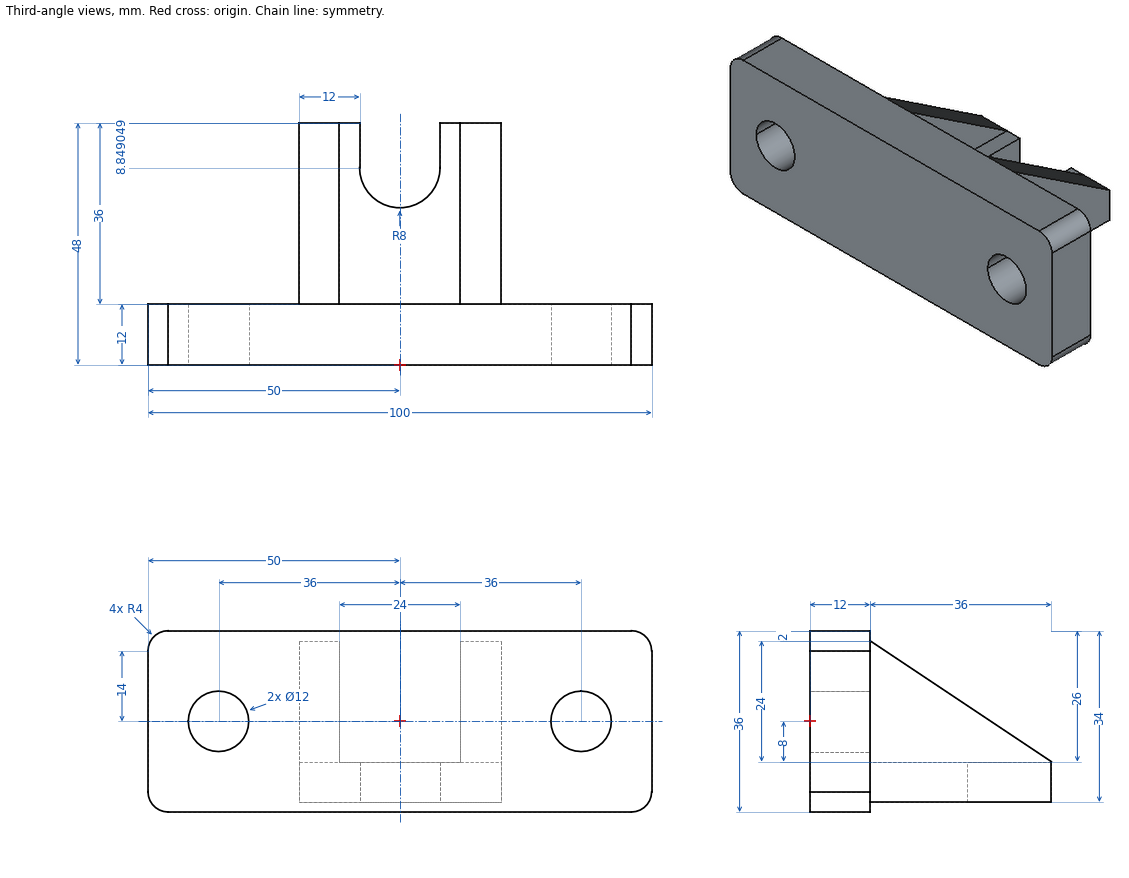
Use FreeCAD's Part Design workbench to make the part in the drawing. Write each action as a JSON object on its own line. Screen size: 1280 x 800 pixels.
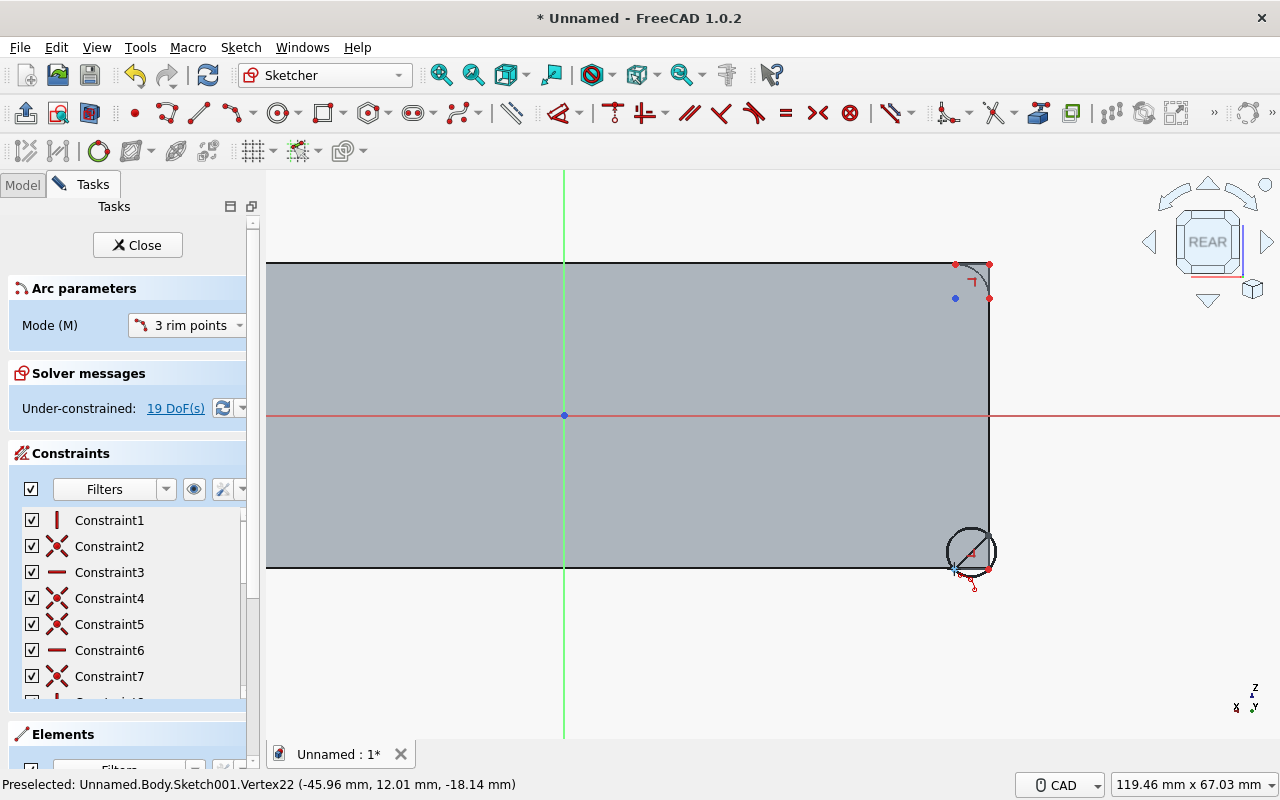
{"action": "scroll", "coordinate": [979, 558], "scroll_direction": "up", "scroll_amount": 3}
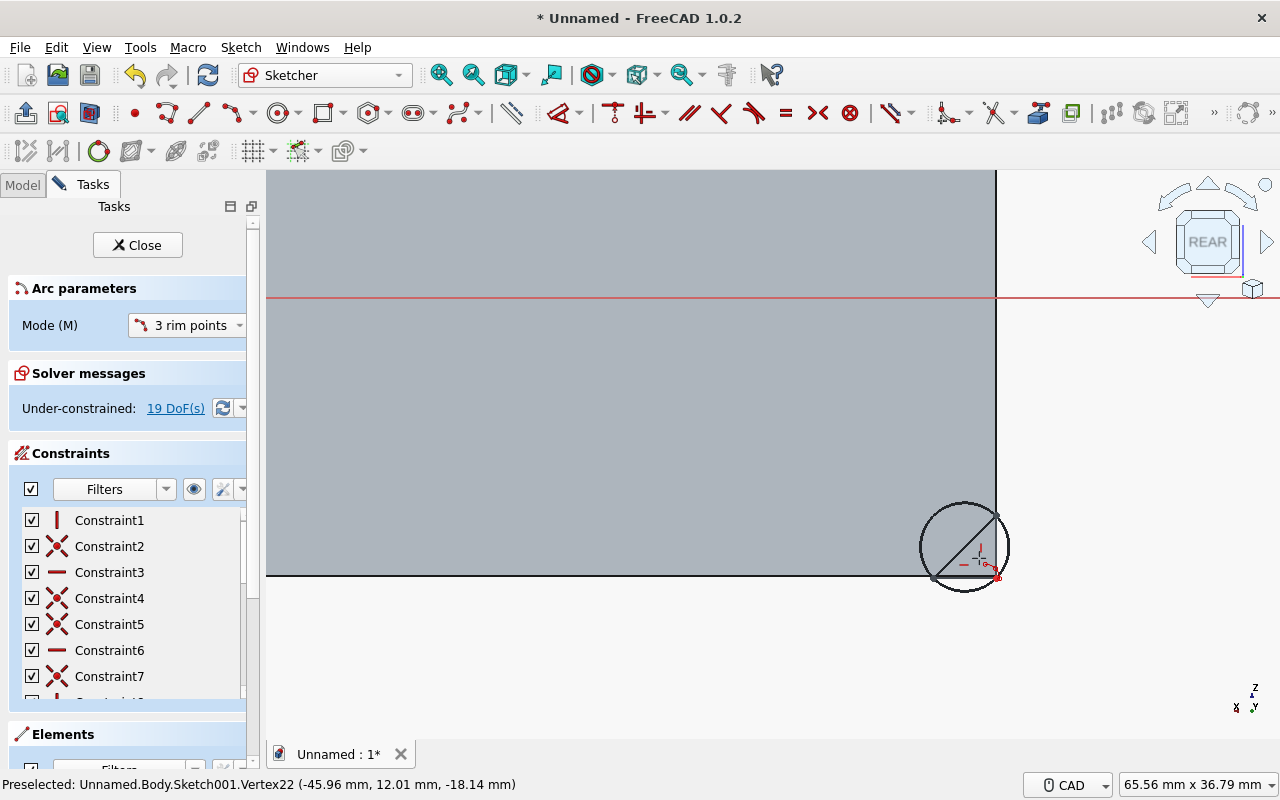
{"action": "left_click", "coordinate": [978, 558]}
{"action": "key", "text": "Escape"}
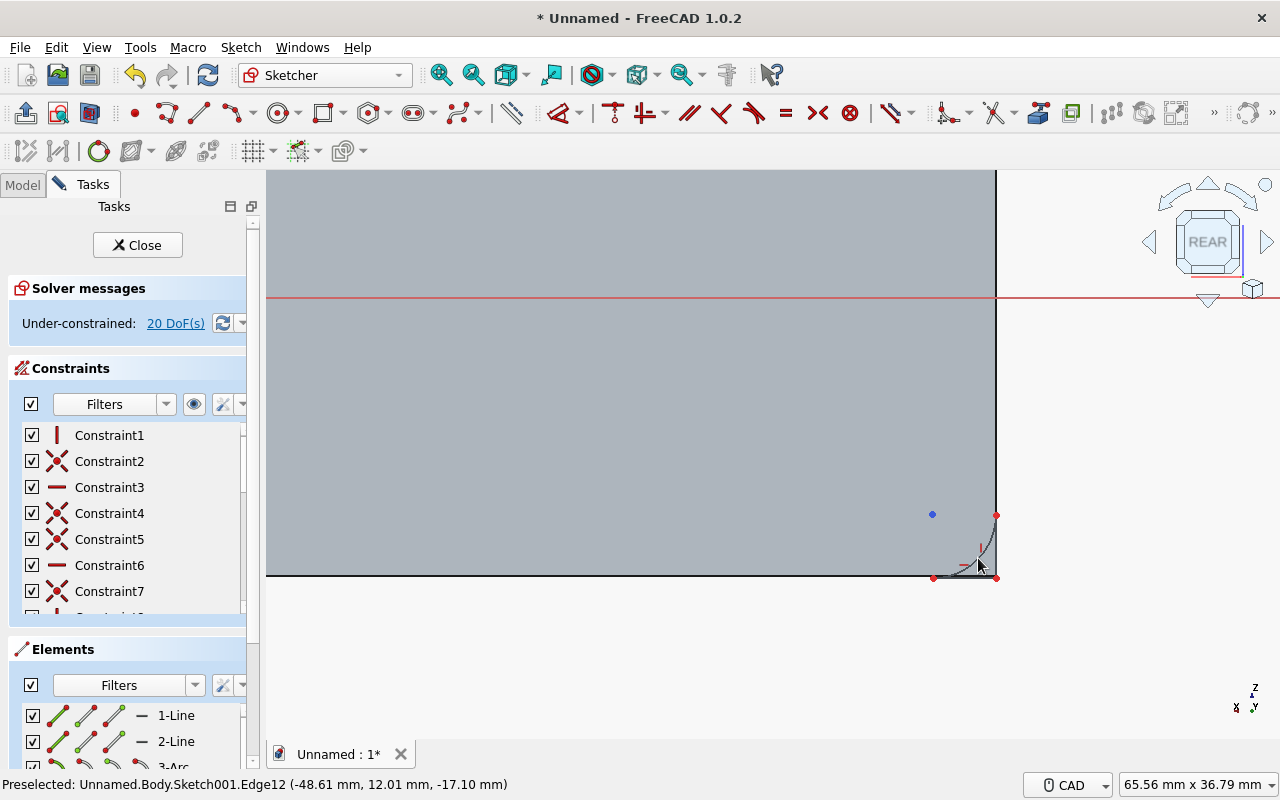
{"action": "scroll", "coordinate": [985, 546], "scroll_direction": "down", "scroll_amount": 5}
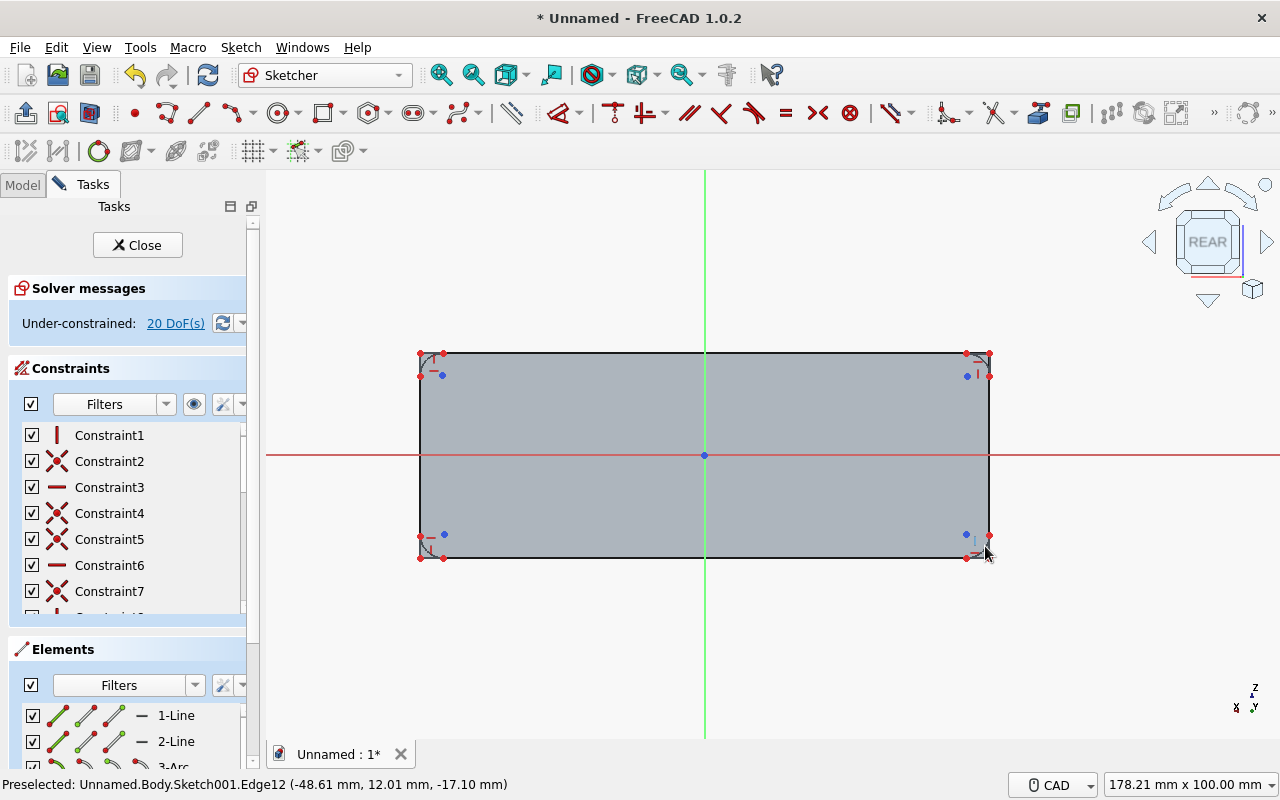
{"action": "scroll", "coordinate": [990, 361], "scroll_direction": "up", "scroll_amount": 6}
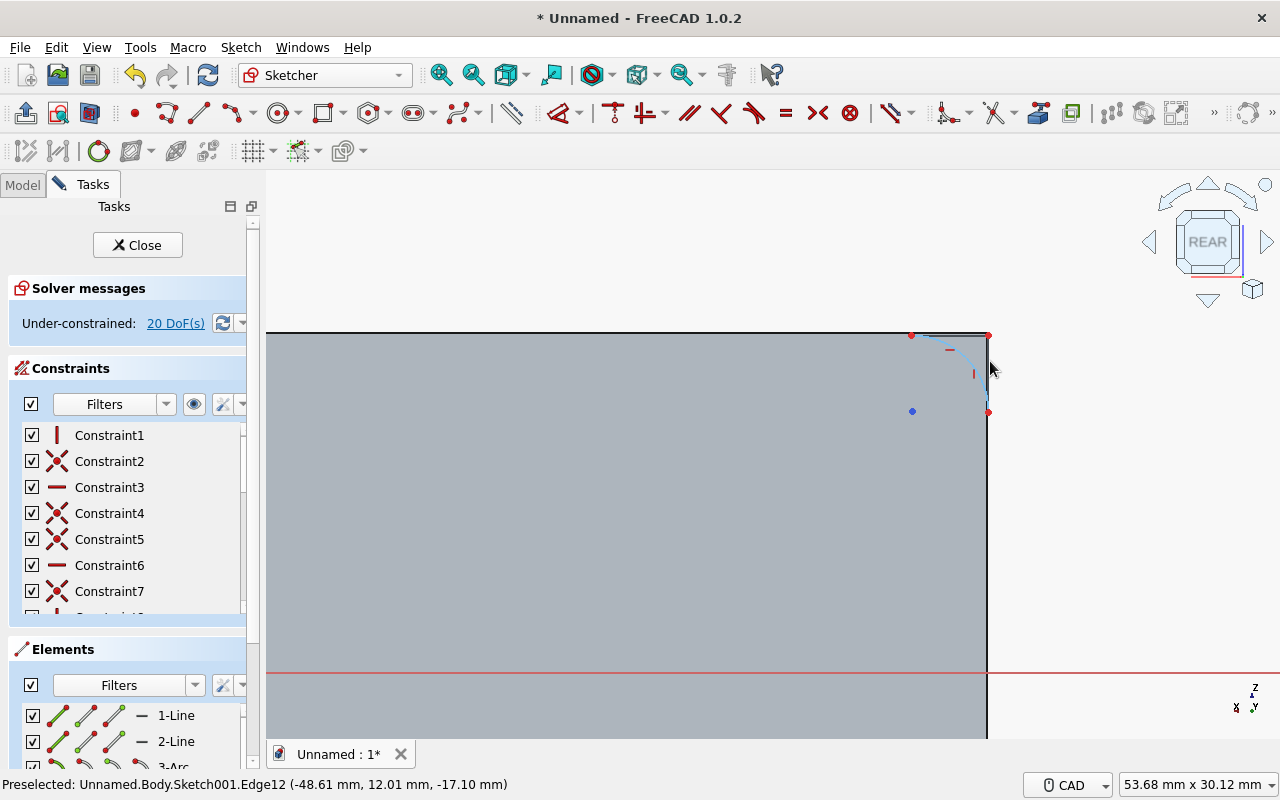
{"action": "left_click", "coordinate": [988, 359]}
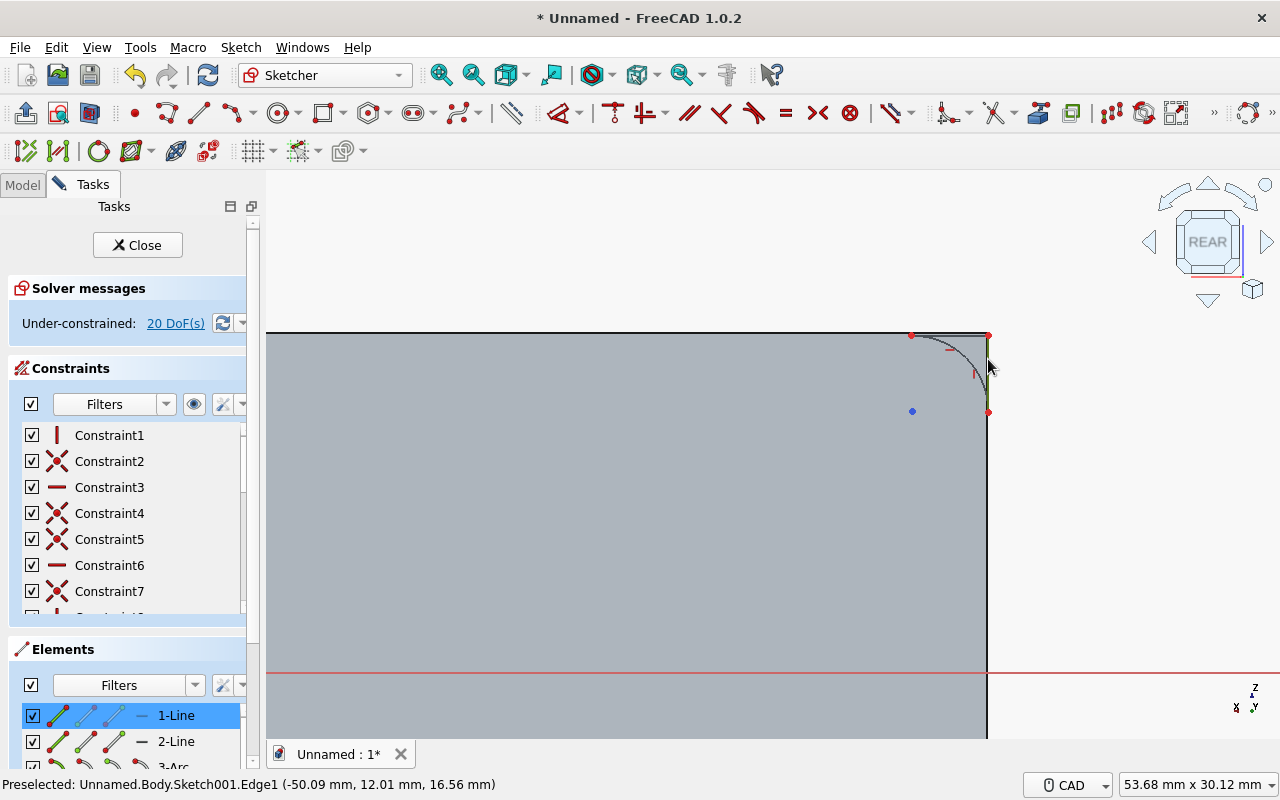
{"action": "left_click", "coordinate": [966, 358]}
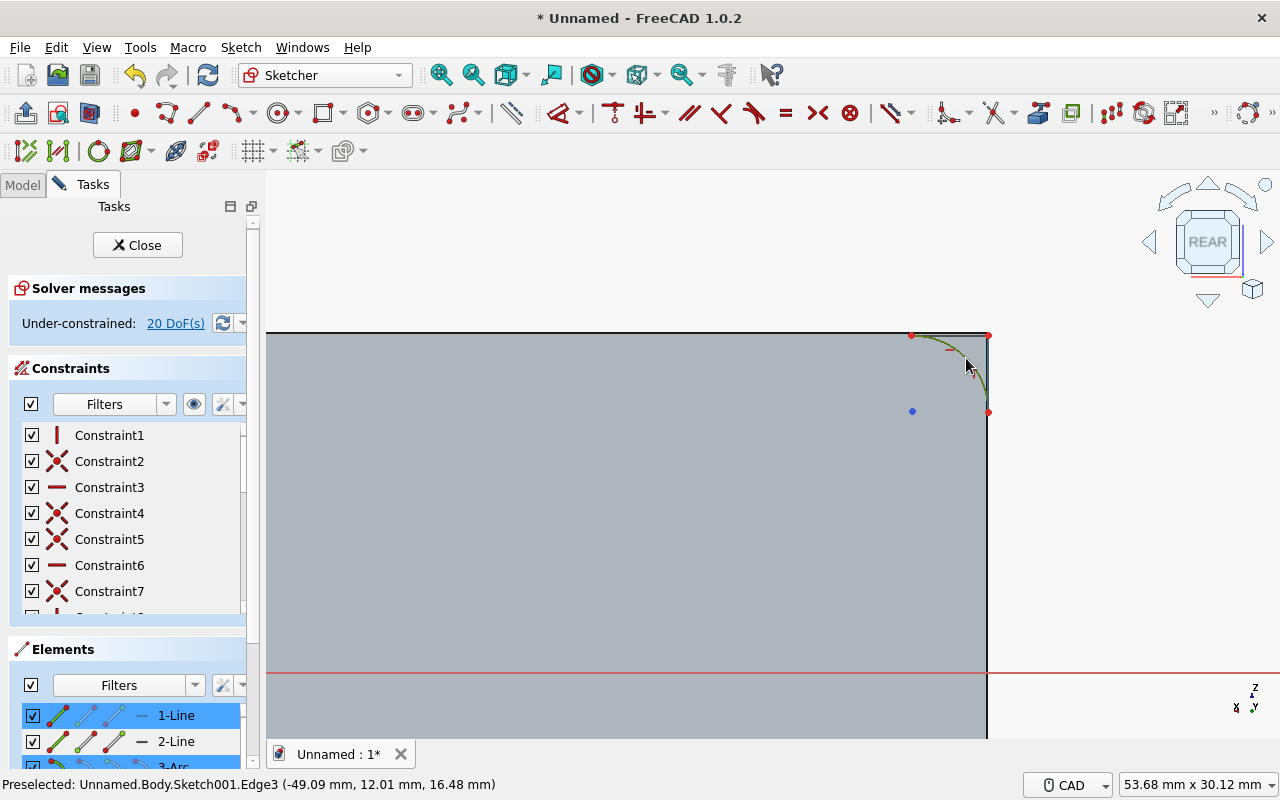
{"action": "left_click", "coordinate": [754, 114]}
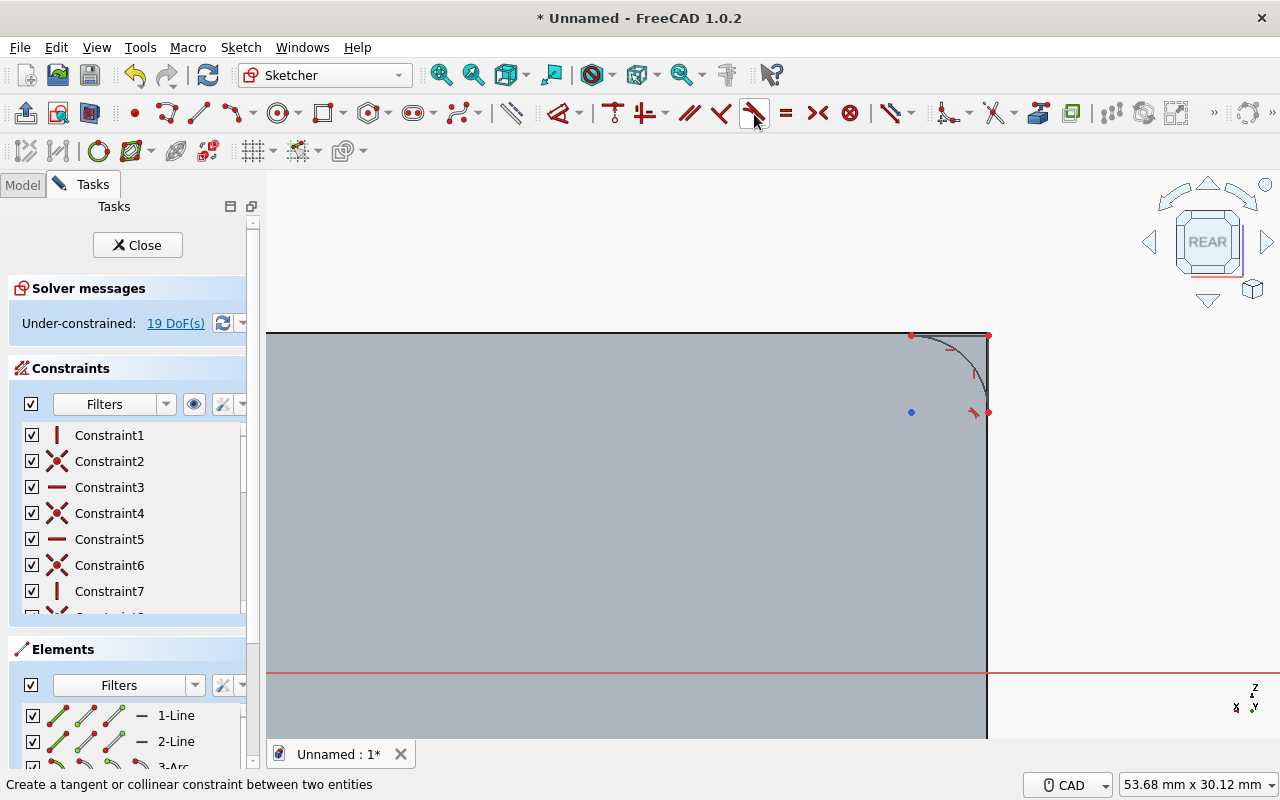
{"action": "left_click", "coordinate": [965, 336]}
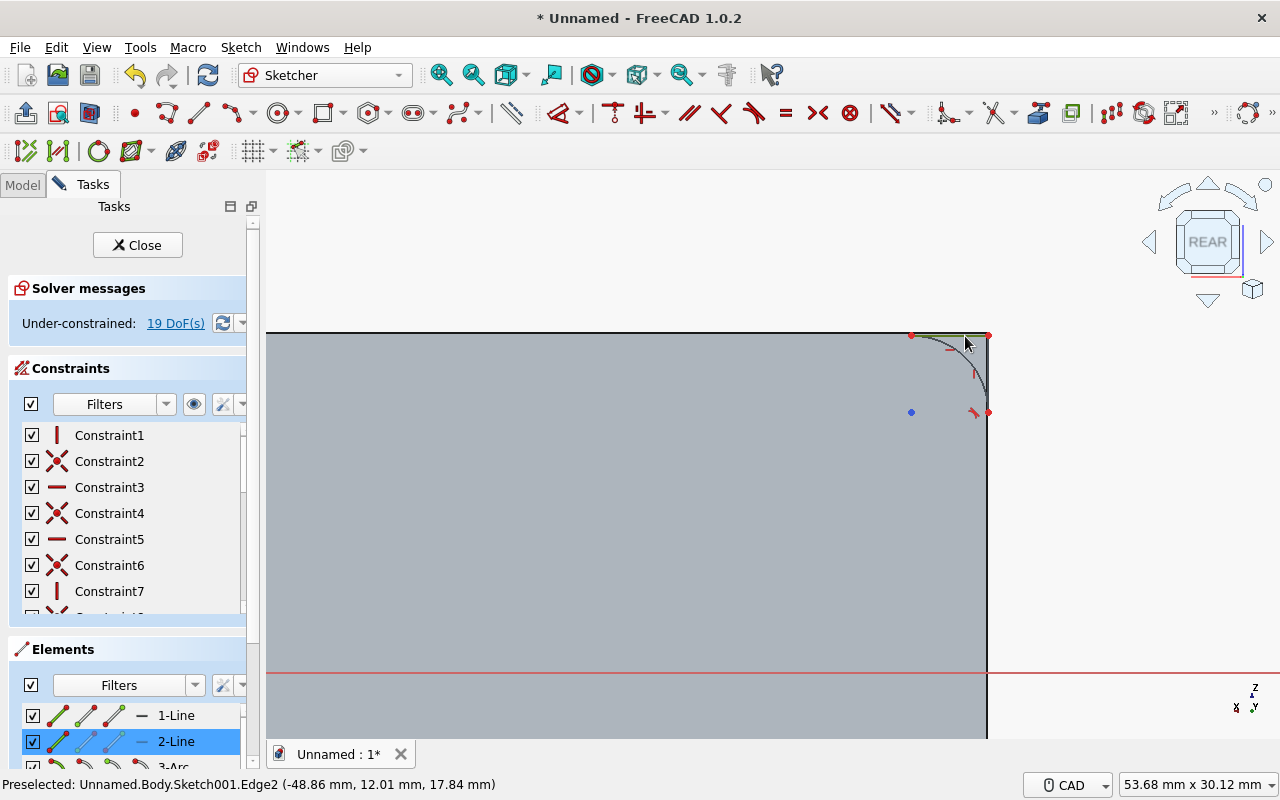
{"action": "left_click", "coordinate": [966, 358]}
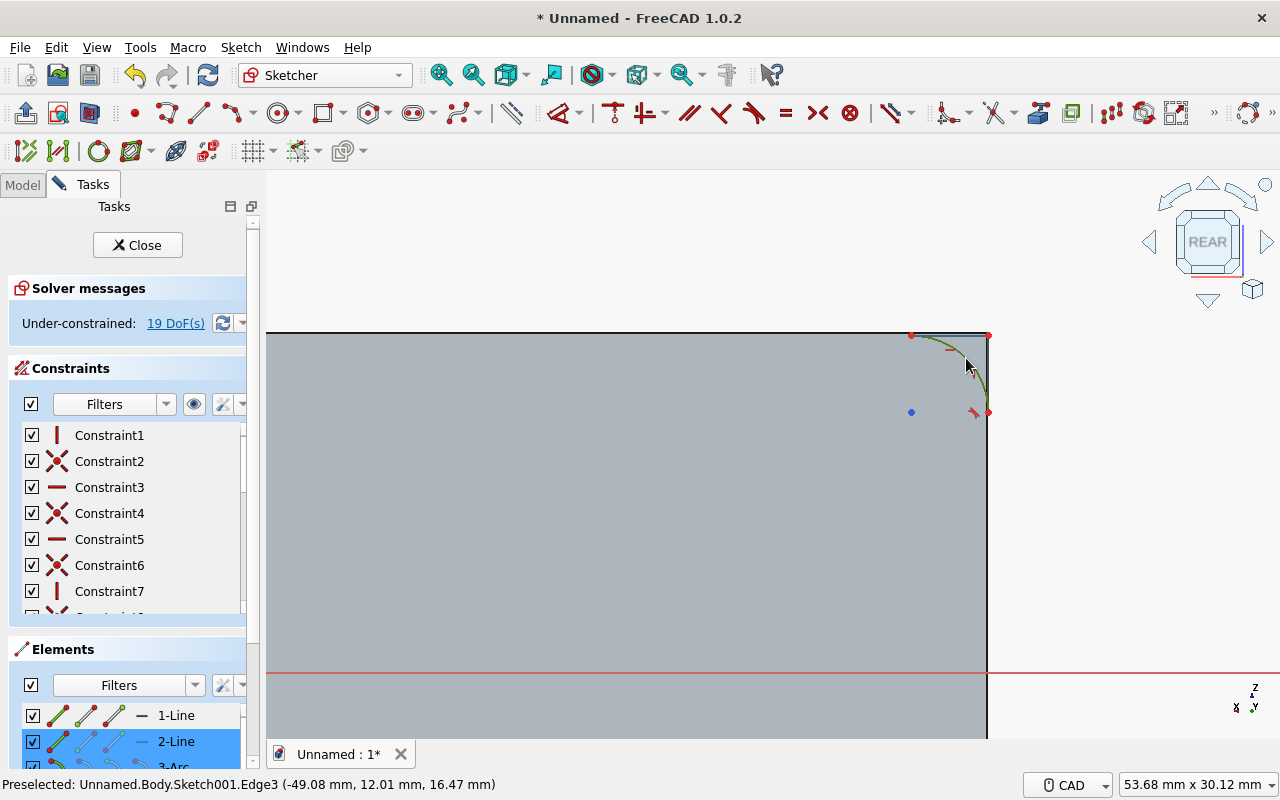
{"action": "left_click", "coordinate": [754, 114]}